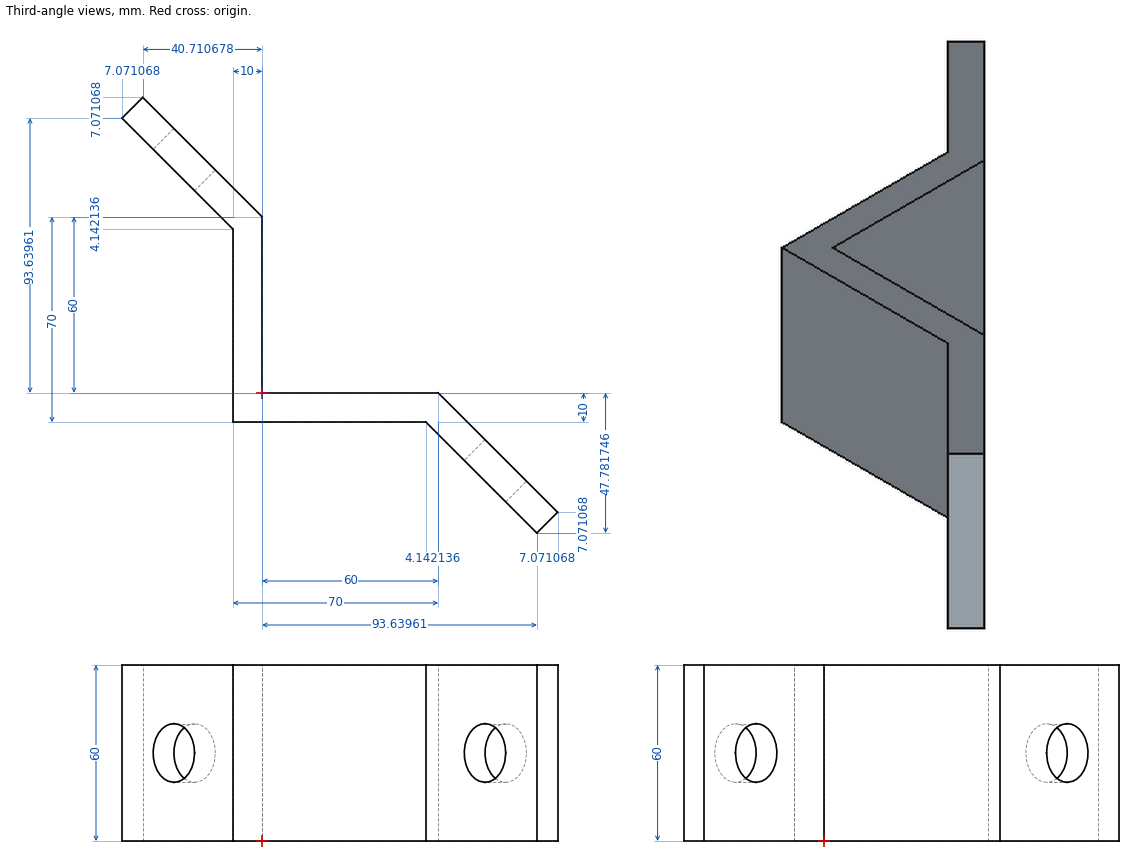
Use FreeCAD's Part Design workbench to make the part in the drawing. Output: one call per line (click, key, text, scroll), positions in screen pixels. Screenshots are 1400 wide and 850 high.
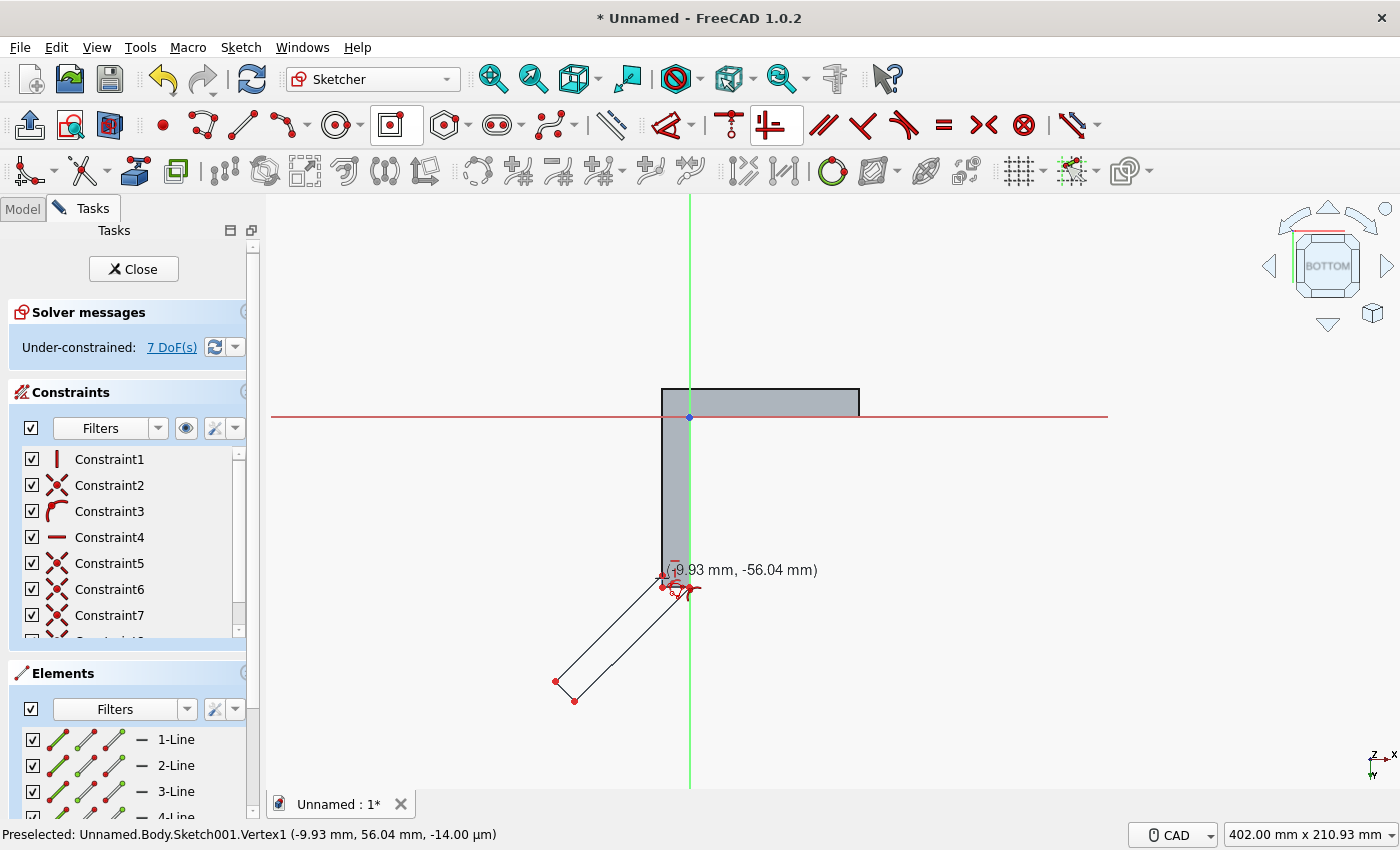
click(848, 389)
click(954, 283)
click(974, 302)
click(859, 417)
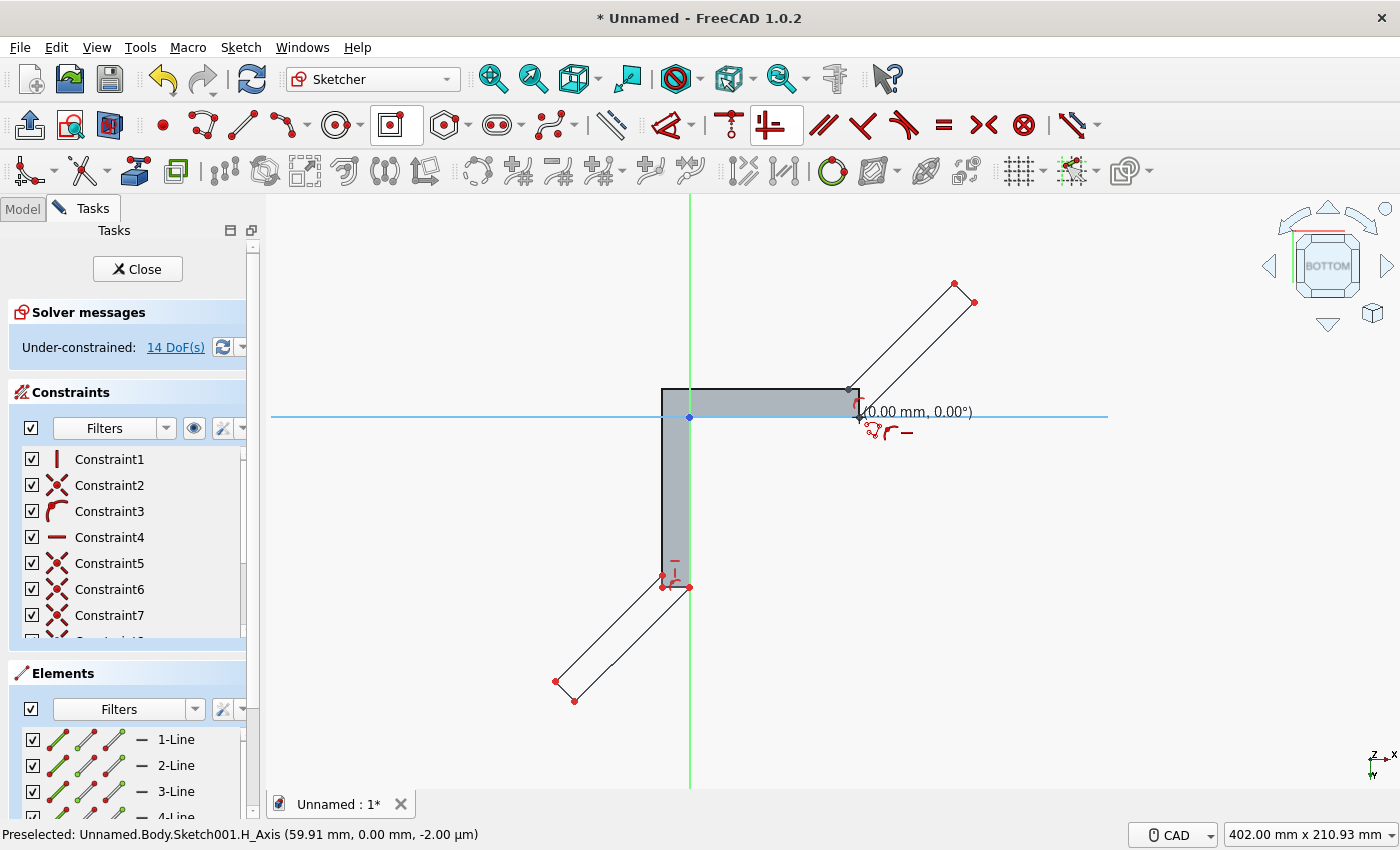
scroll(859, 389, up, 4)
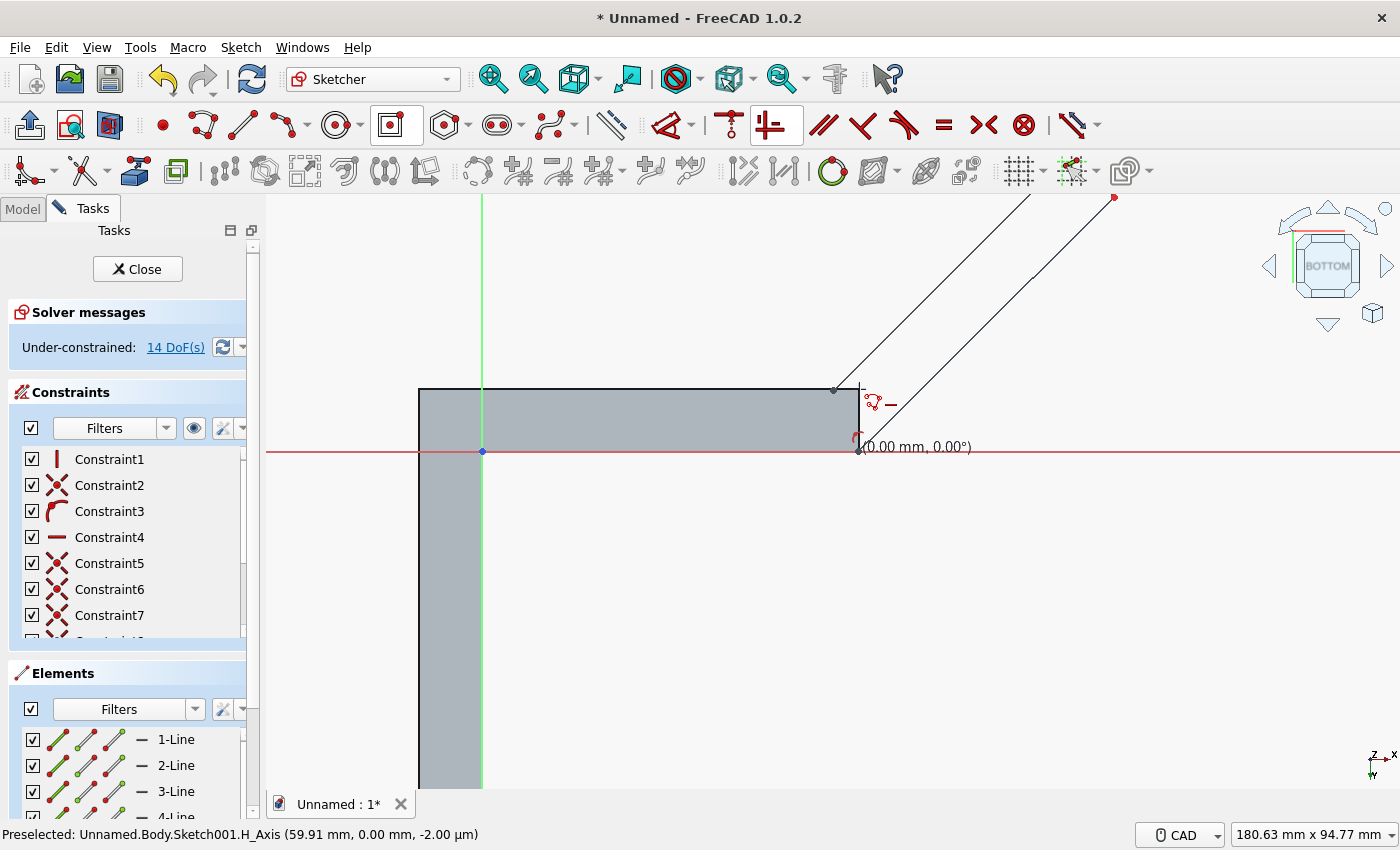
click(858, 389)
click(834, 391)
key(Escape)
key(Escape)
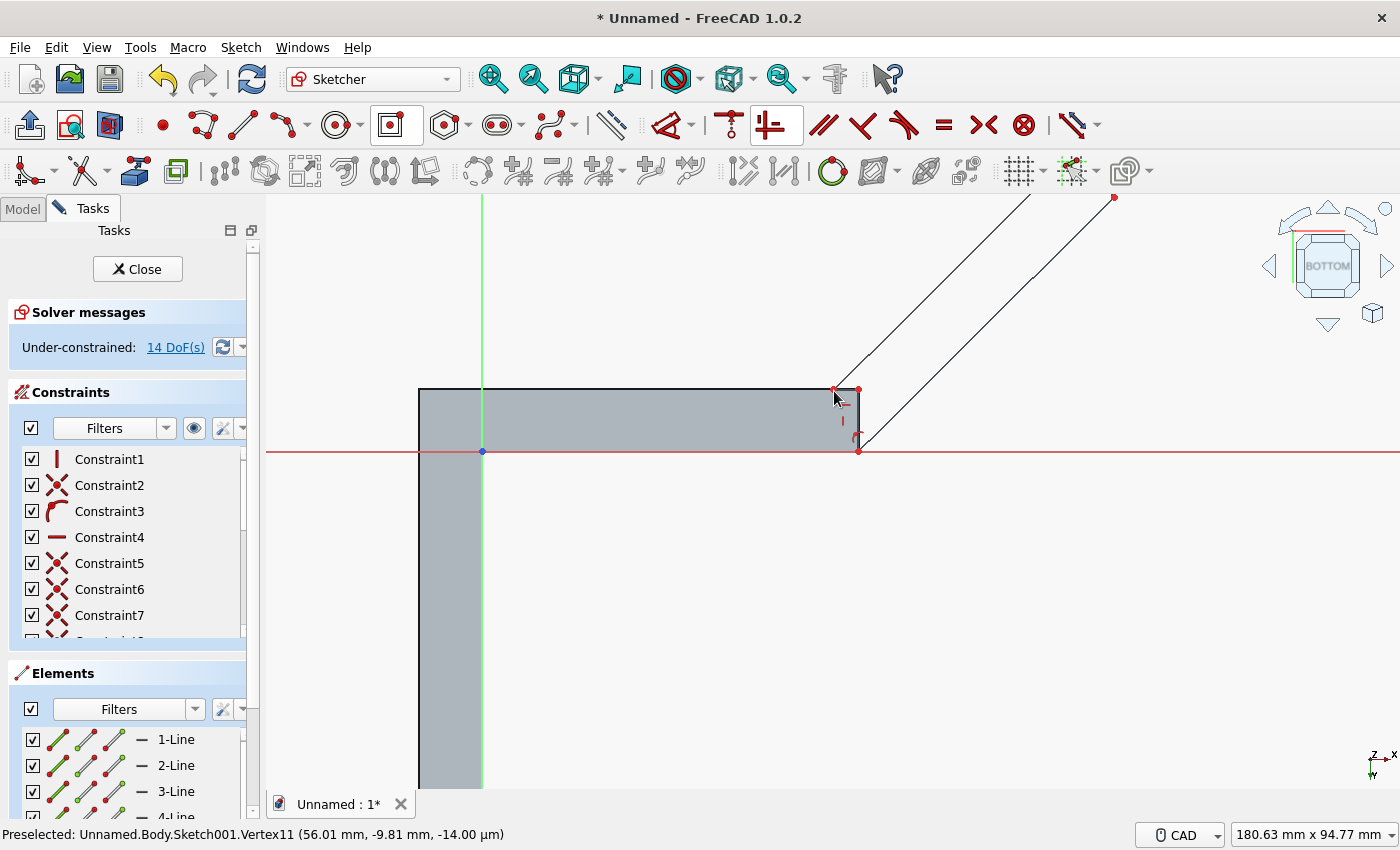
click(666, 126)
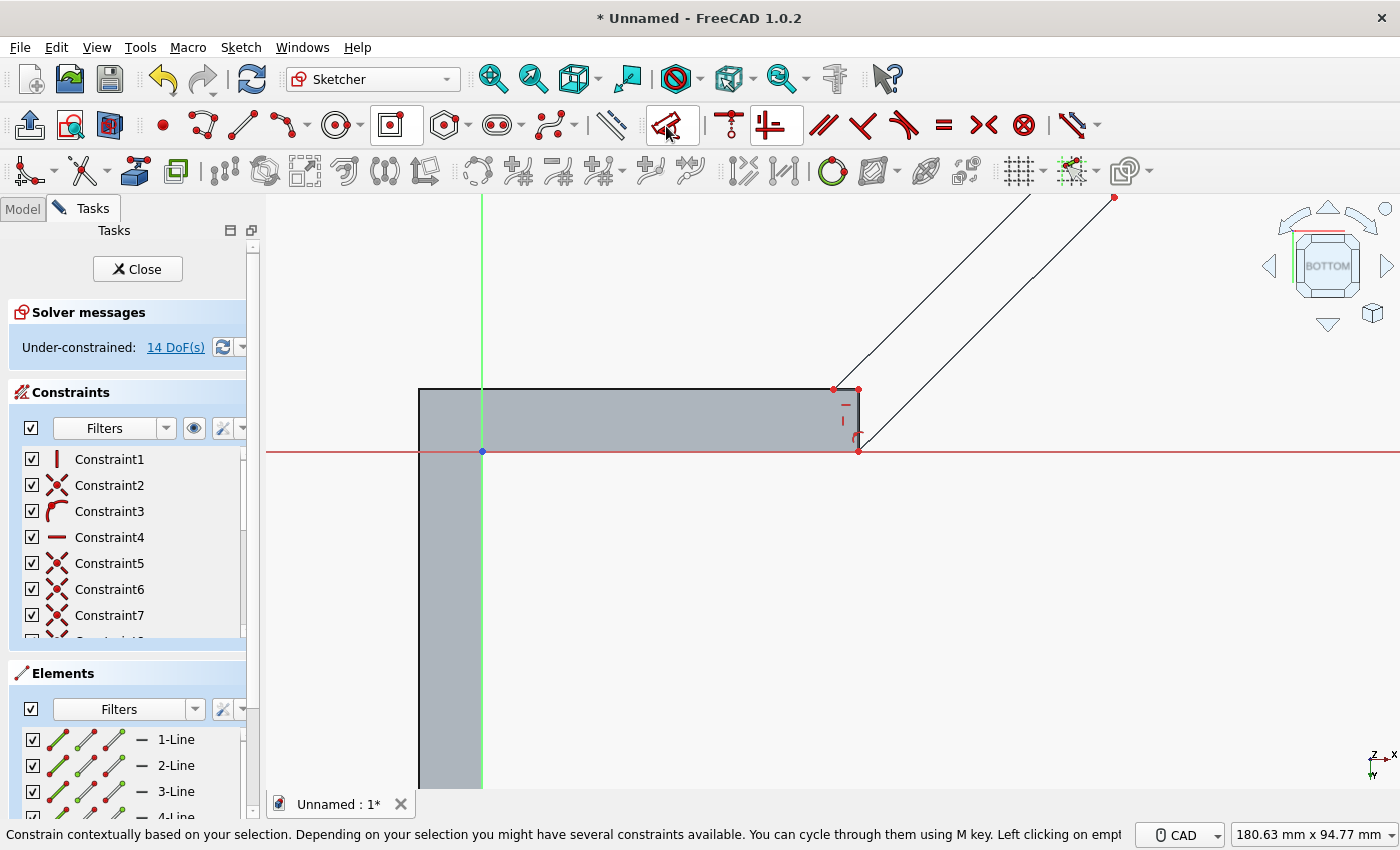
scroll(859, 389, down, 4)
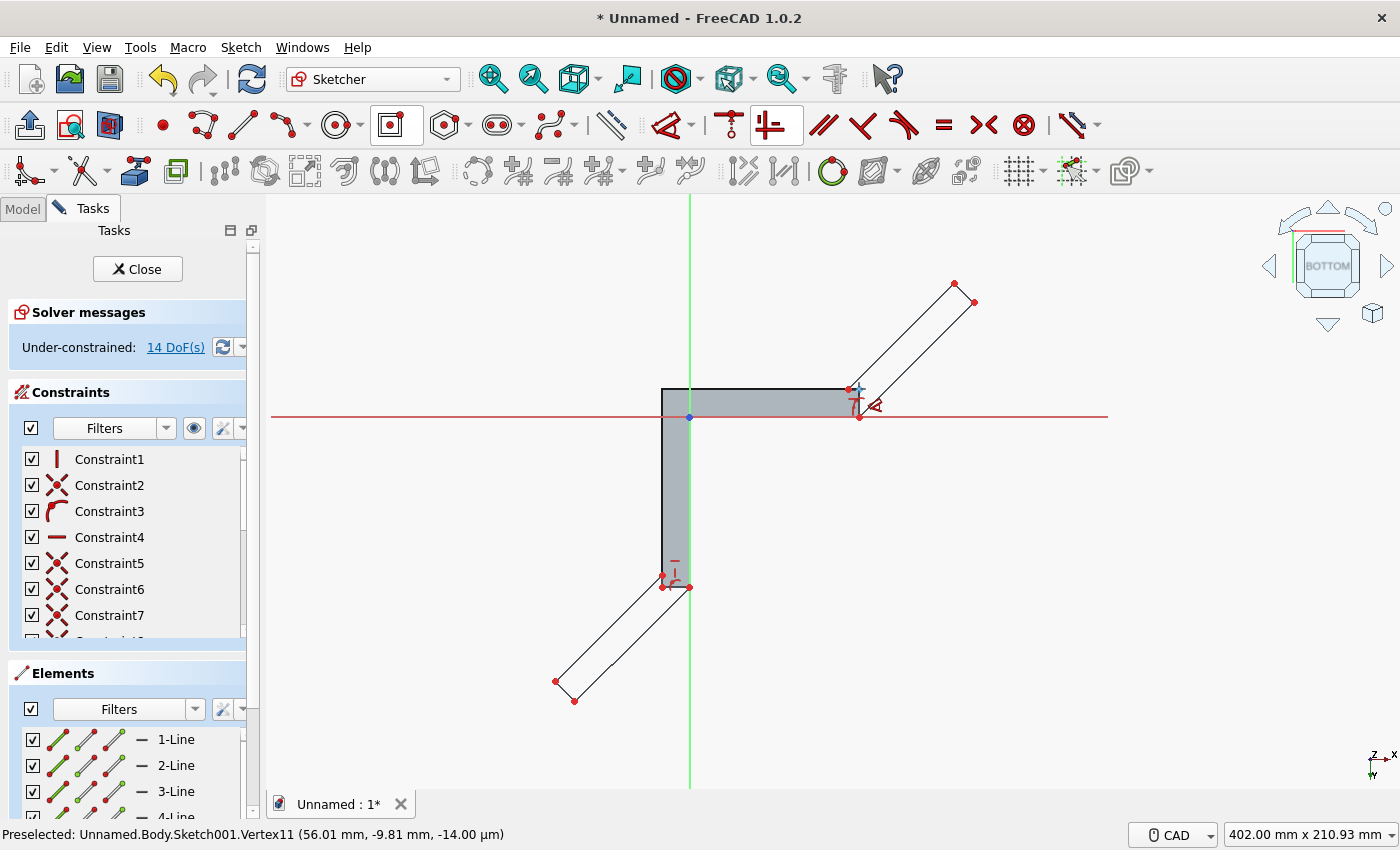
scroll(670, 587, up, 3)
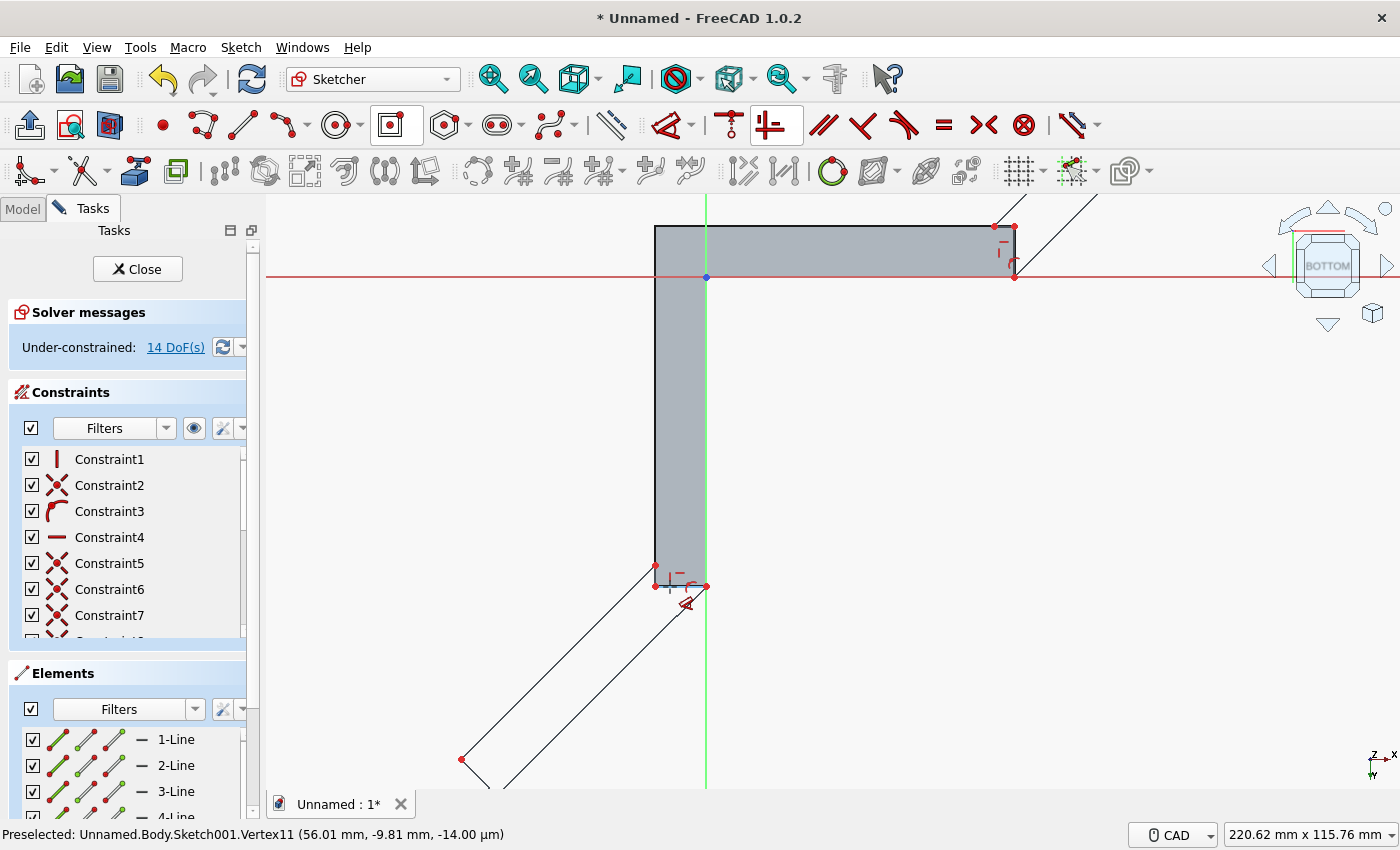
click(670, 587)
click(692, 621)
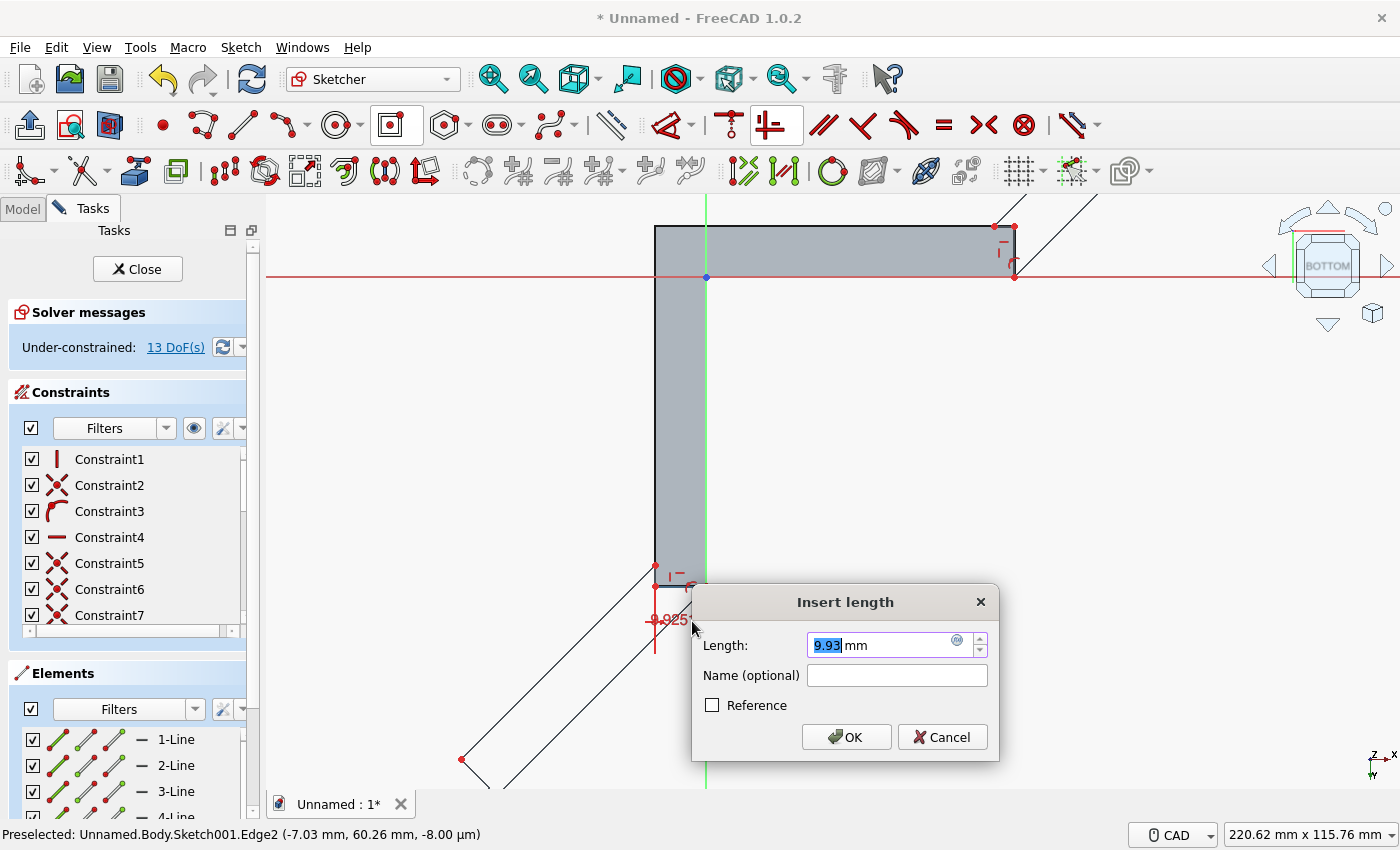
text(10)
key(Return)